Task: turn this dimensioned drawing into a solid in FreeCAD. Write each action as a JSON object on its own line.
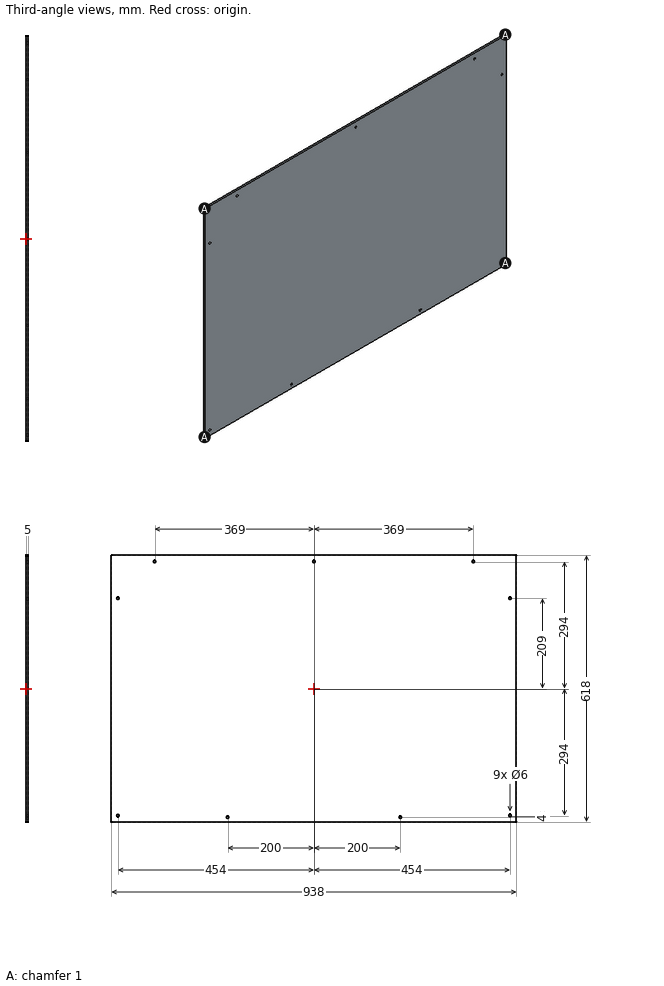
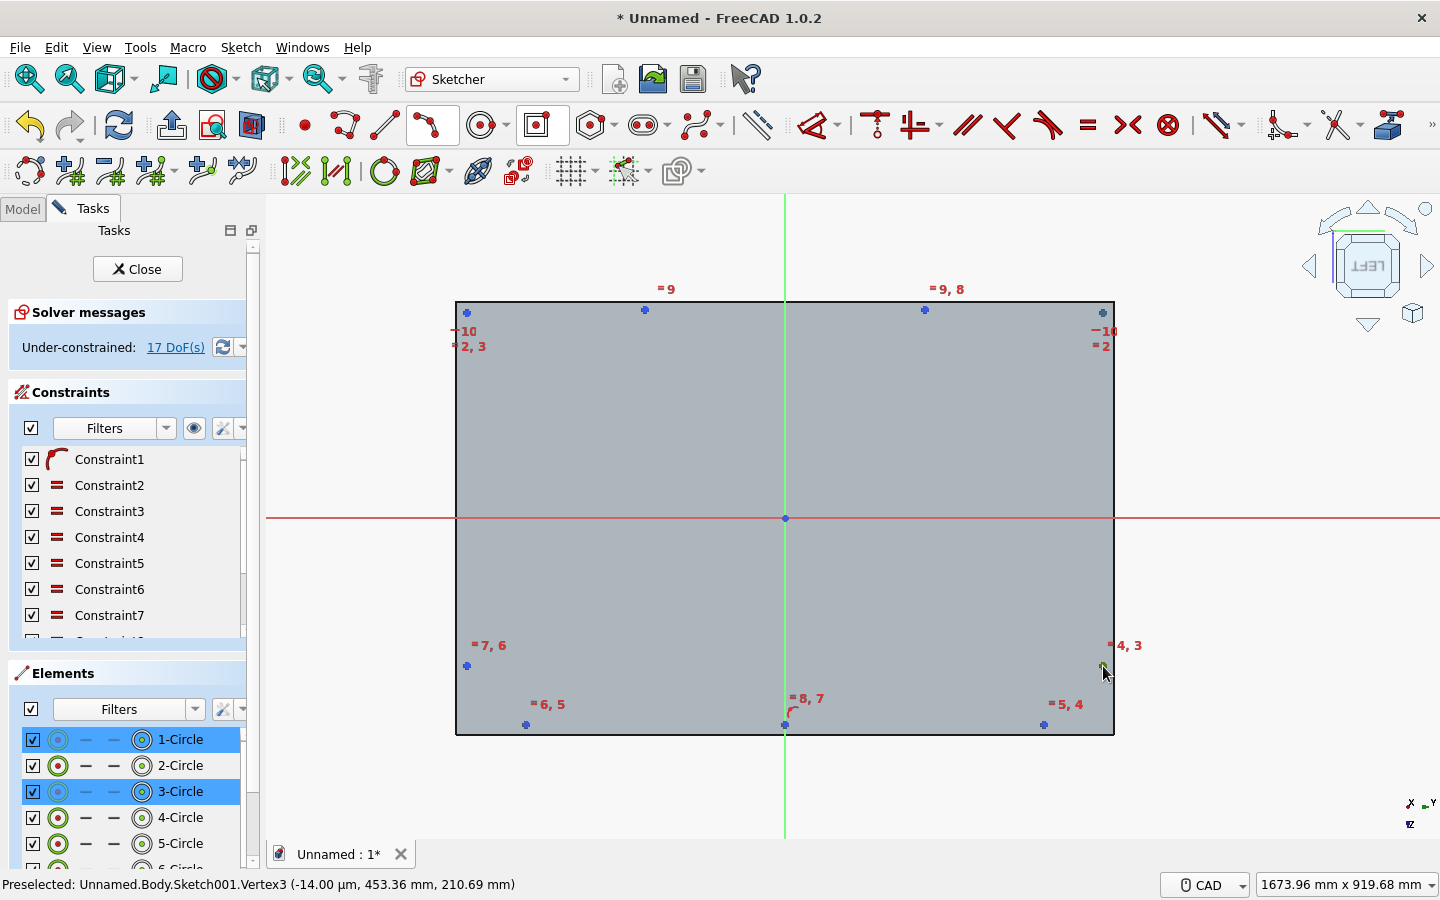
{"action": "key", "text": "v"}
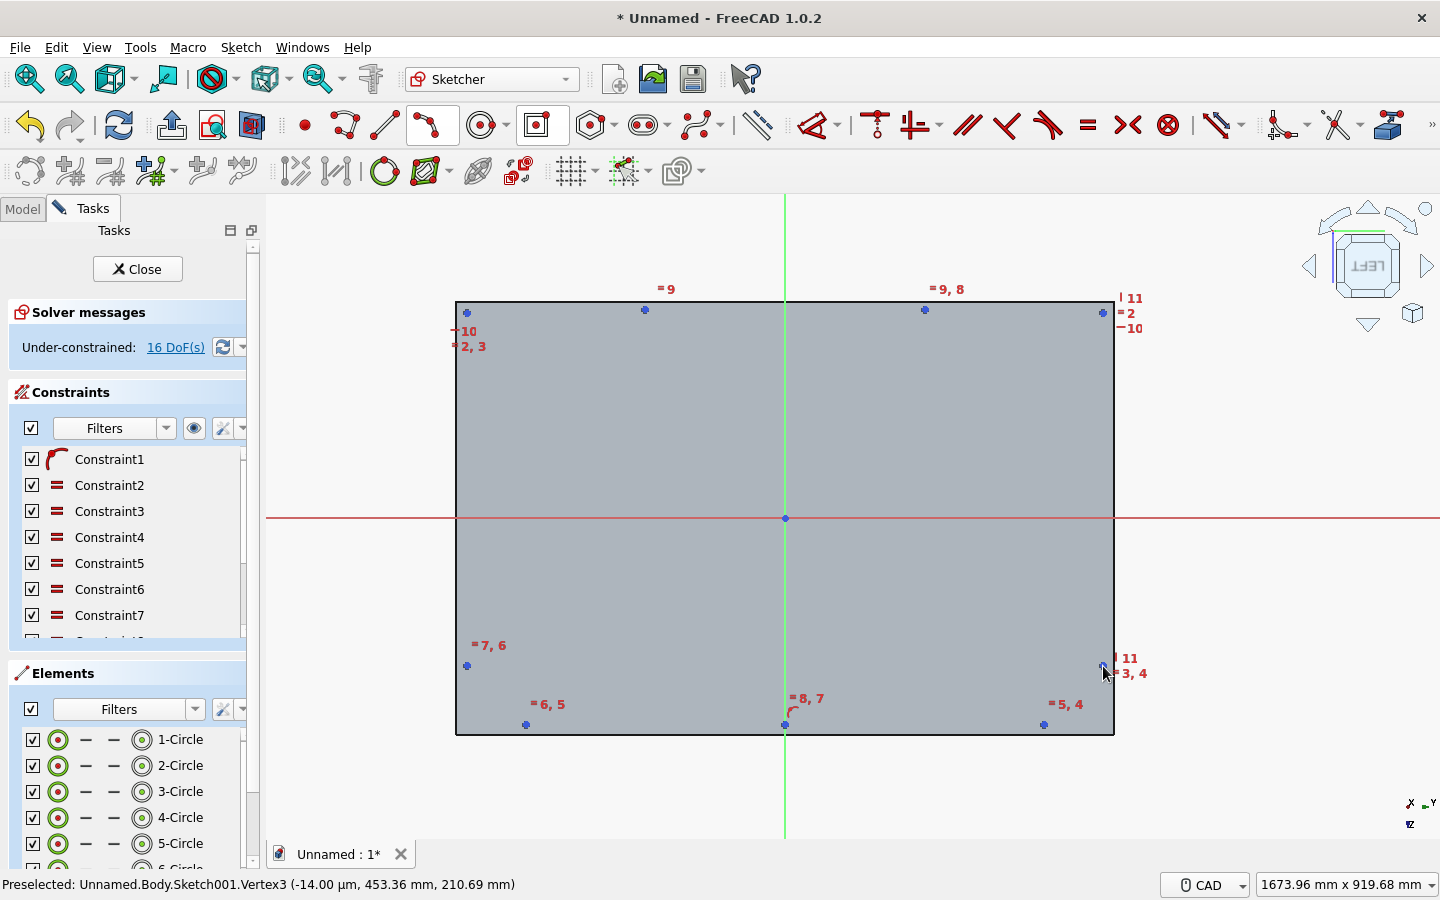
{"action": "left_click", "coordinate": [1044, 725]}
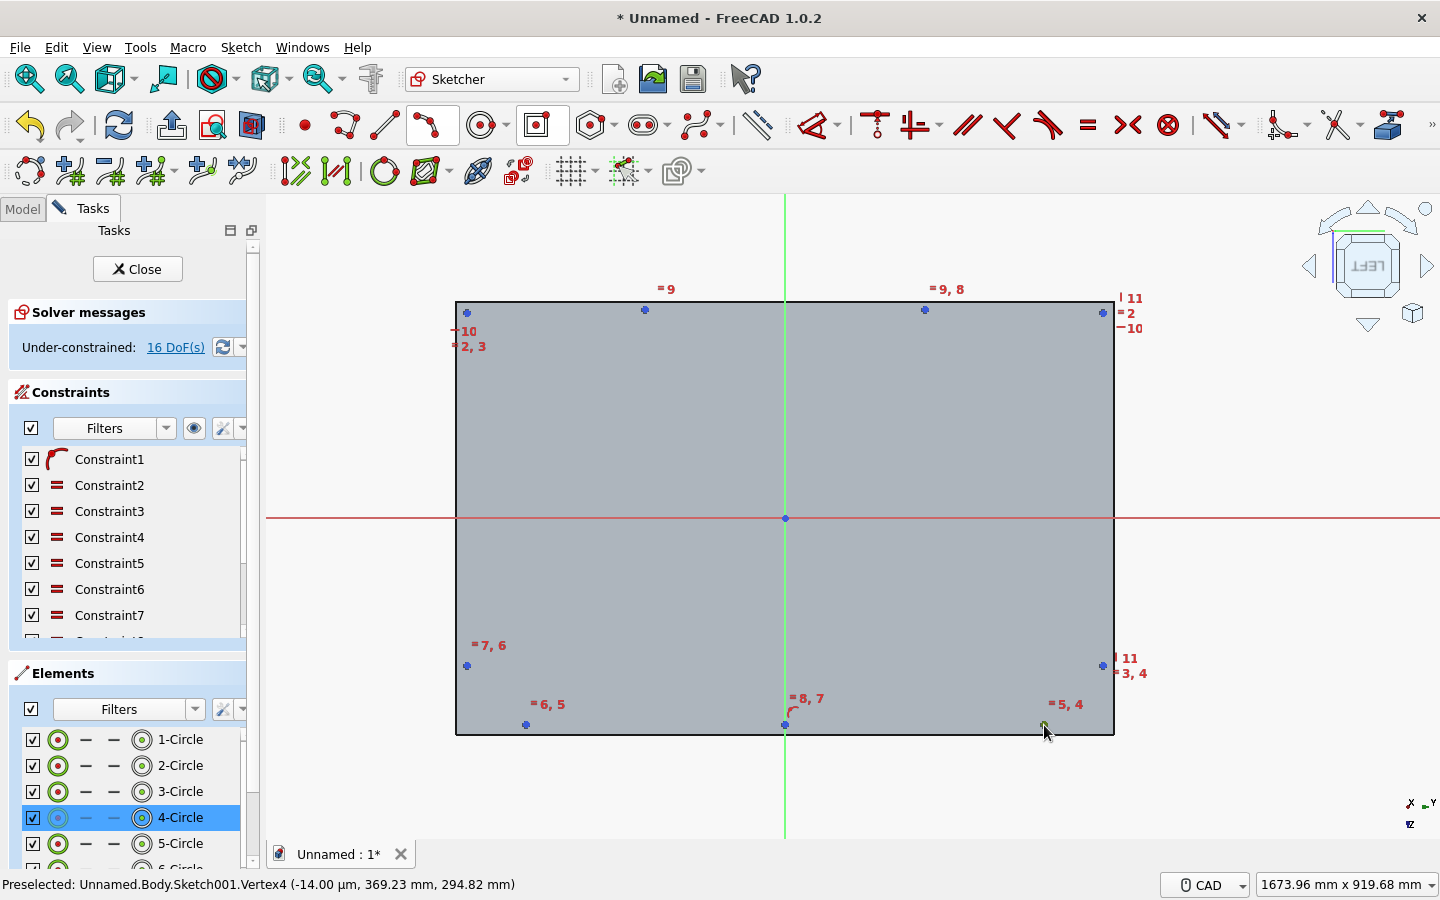
{"action": "left_click", "coordinate": [526, 725]}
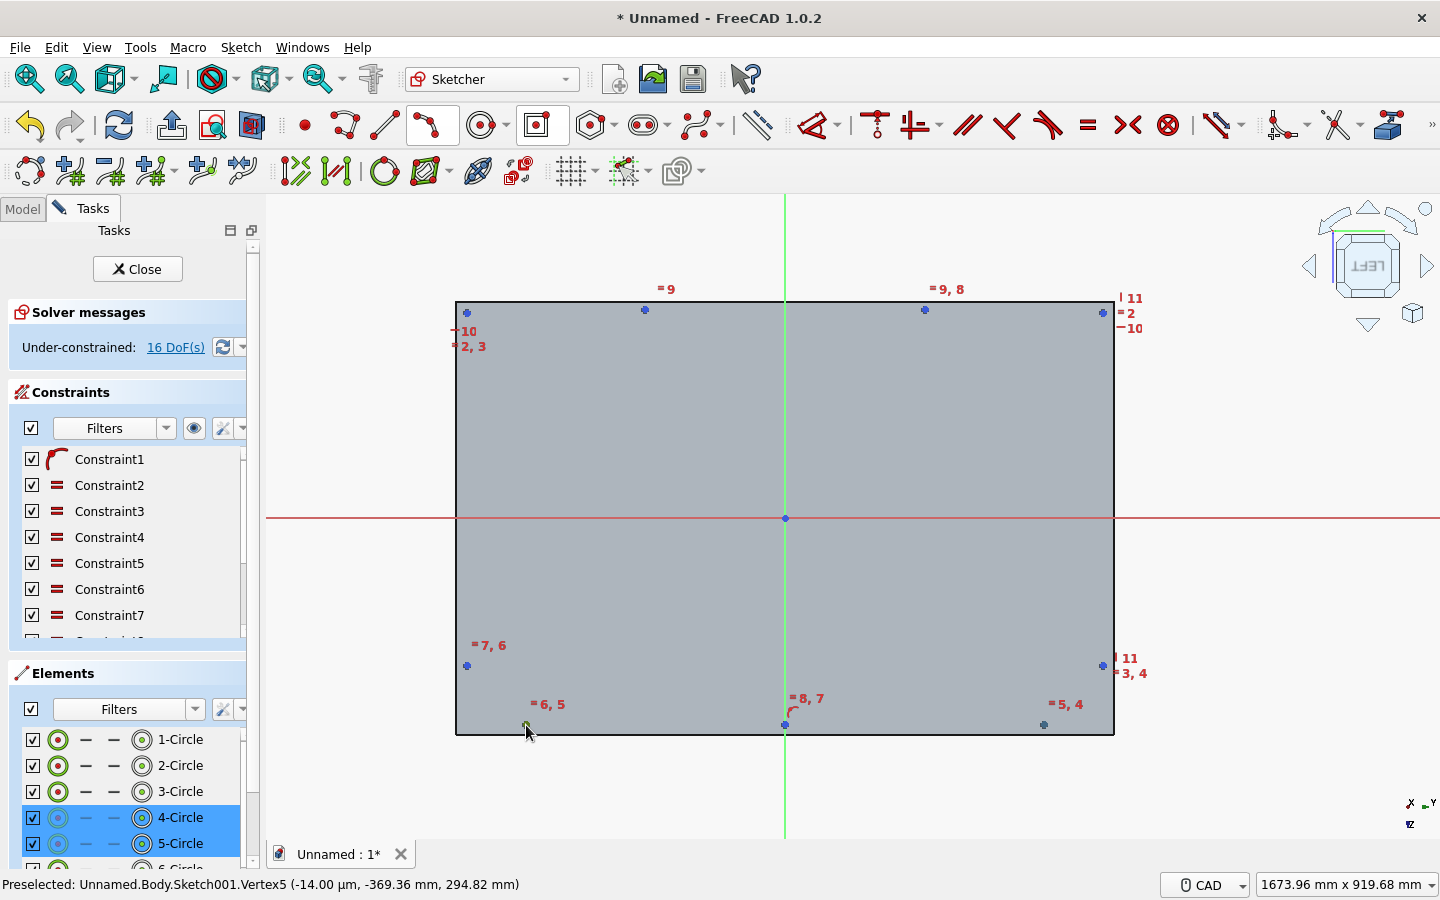
{"action": "key", "text": "h"}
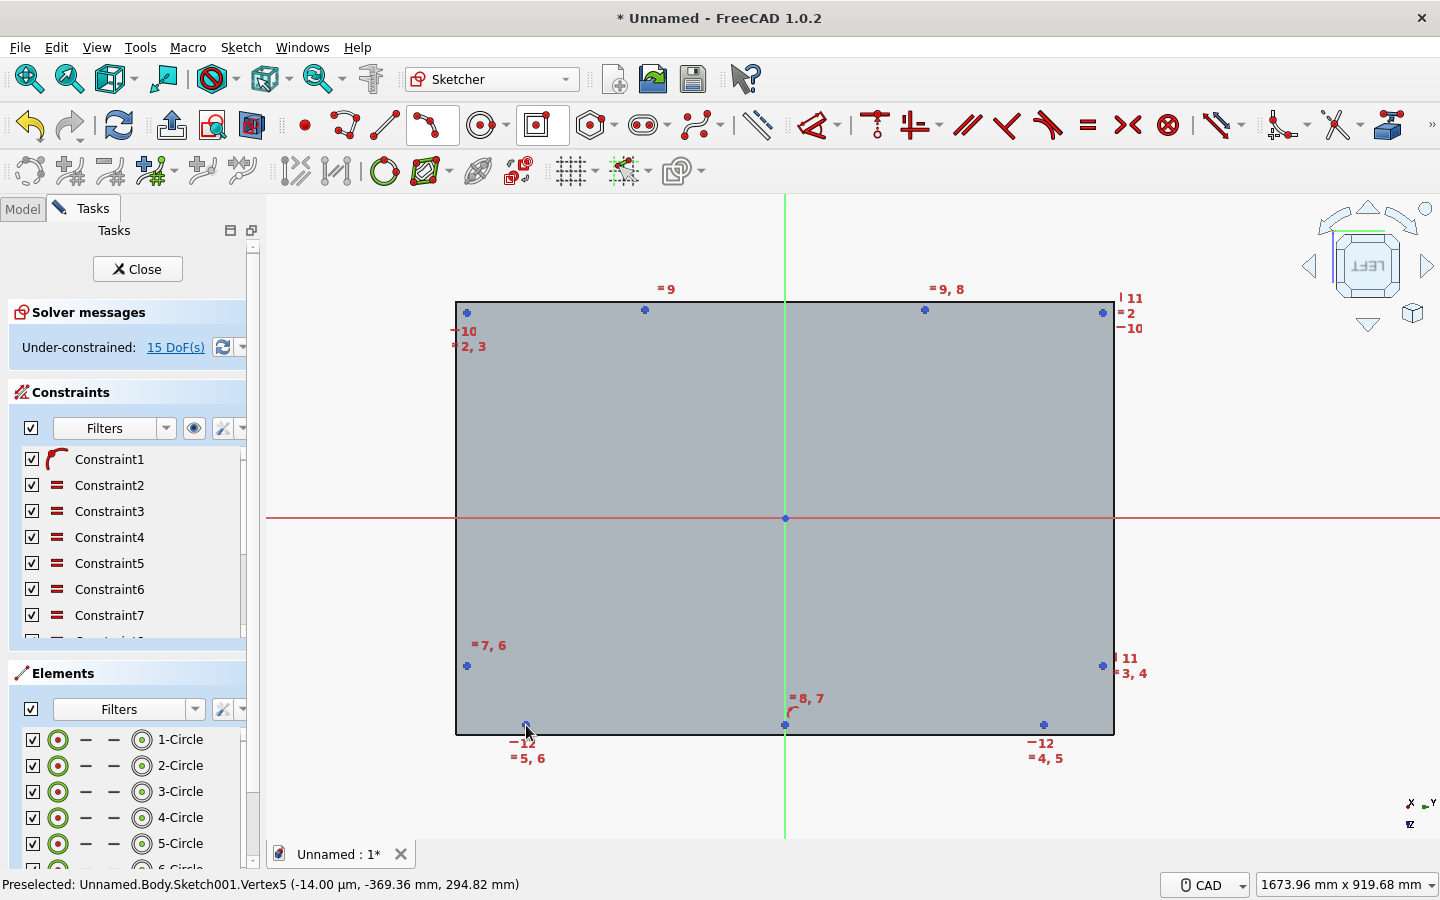
{"action": "left_click", "coordinate": [467, 313]}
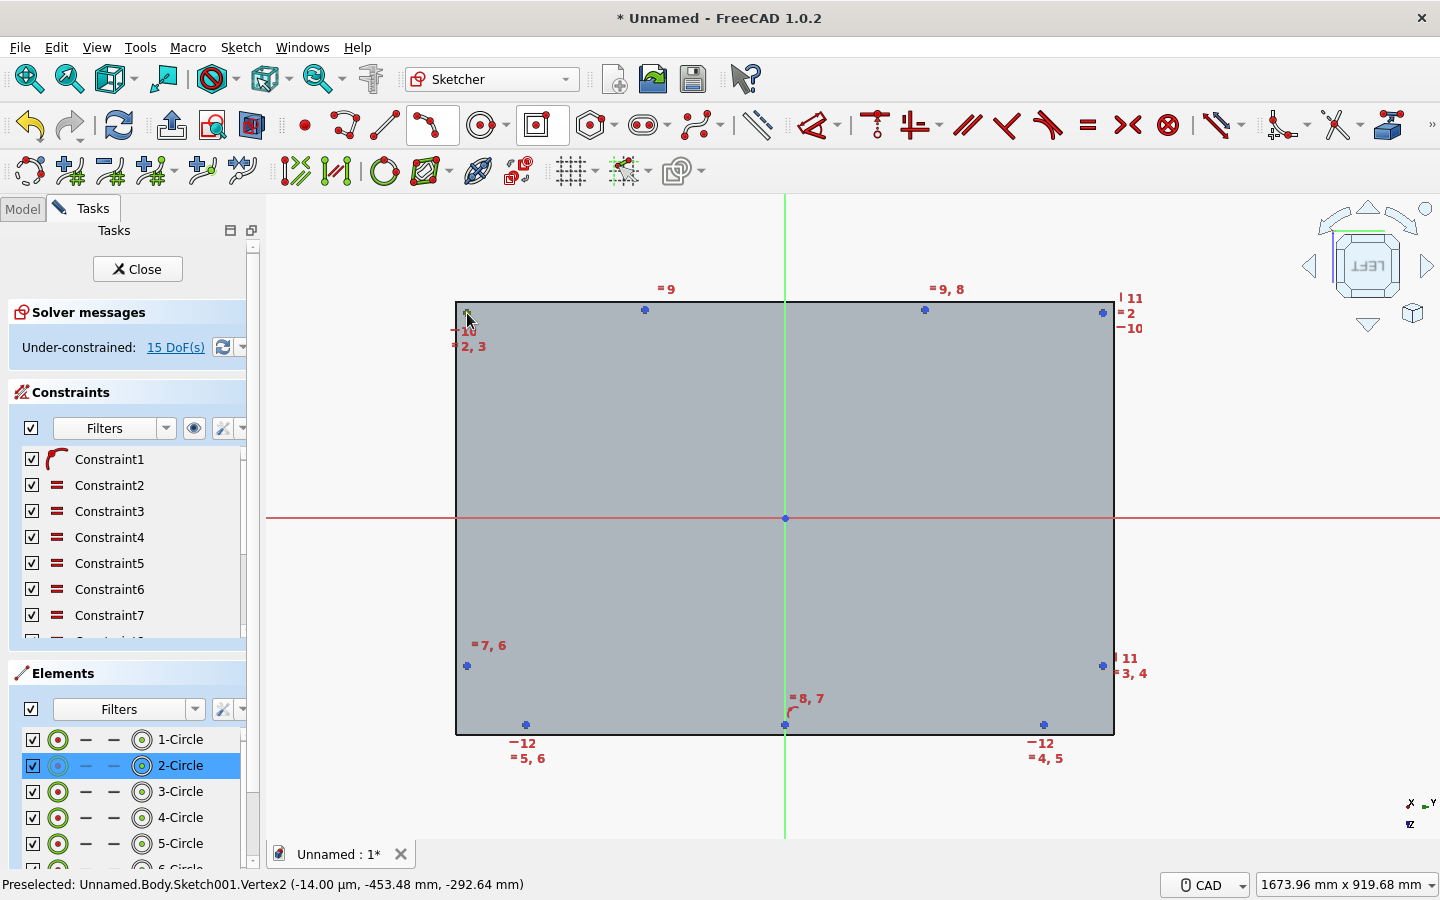
{"action": "left_click", "coordinate": [467, 666]}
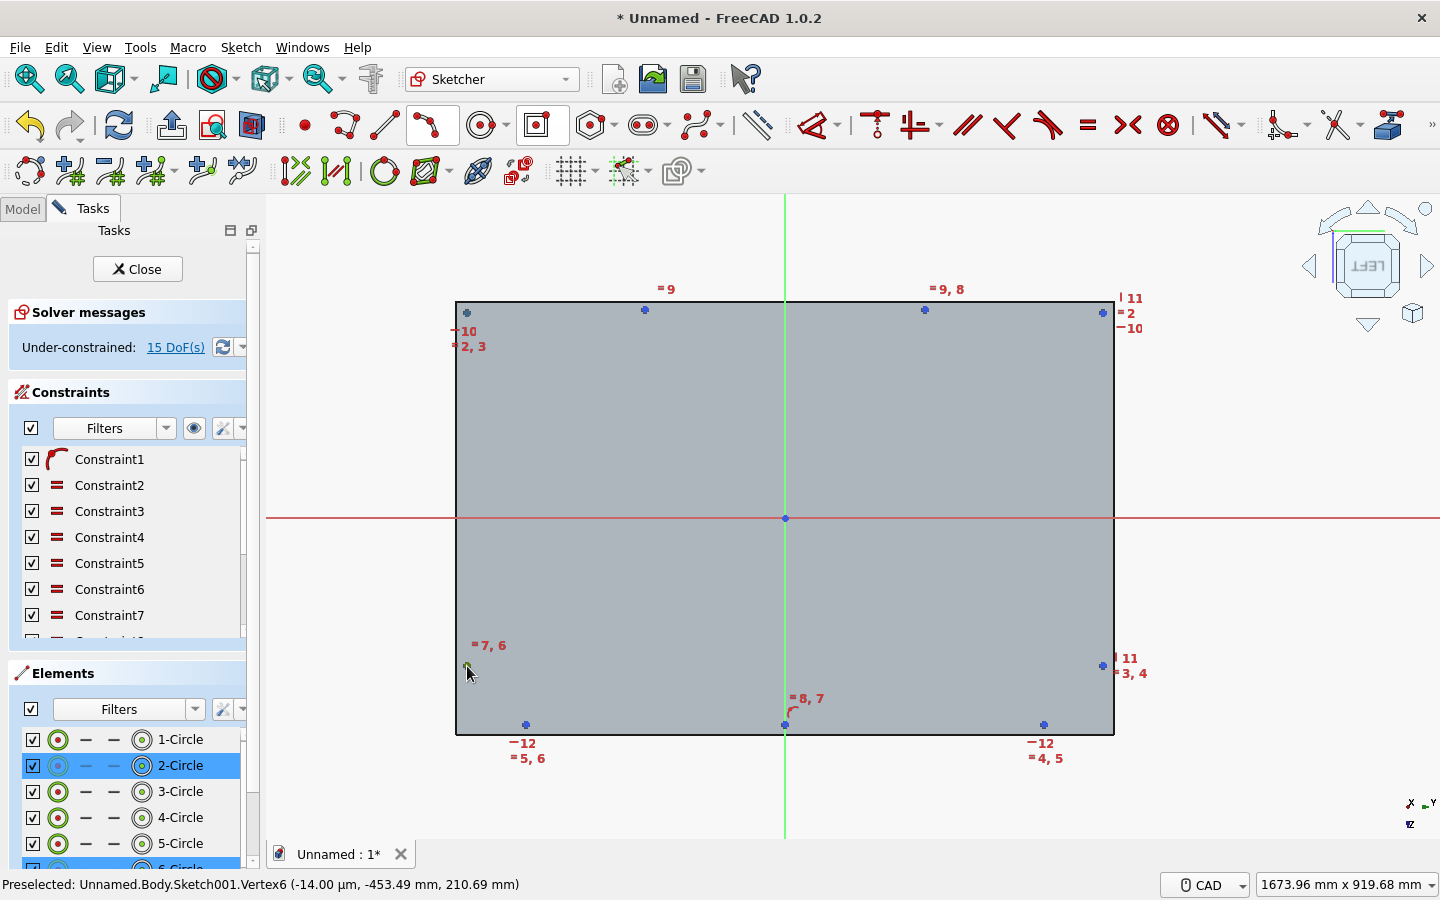
{"action": "left_click", "coordinate": [942, 126]}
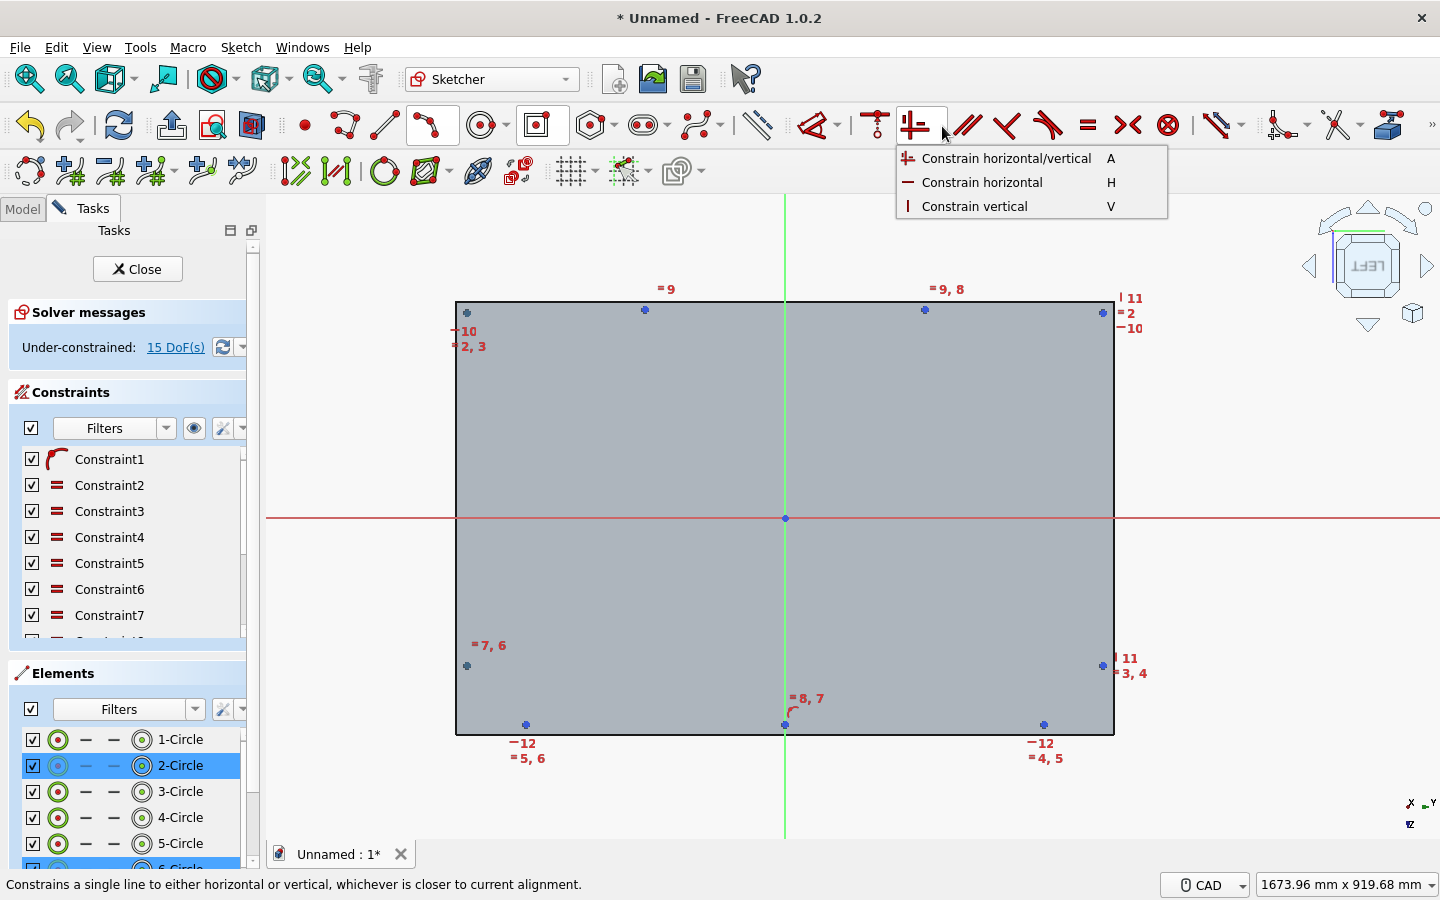
{"action": "left_click", "coordinate": [1032, 206]}